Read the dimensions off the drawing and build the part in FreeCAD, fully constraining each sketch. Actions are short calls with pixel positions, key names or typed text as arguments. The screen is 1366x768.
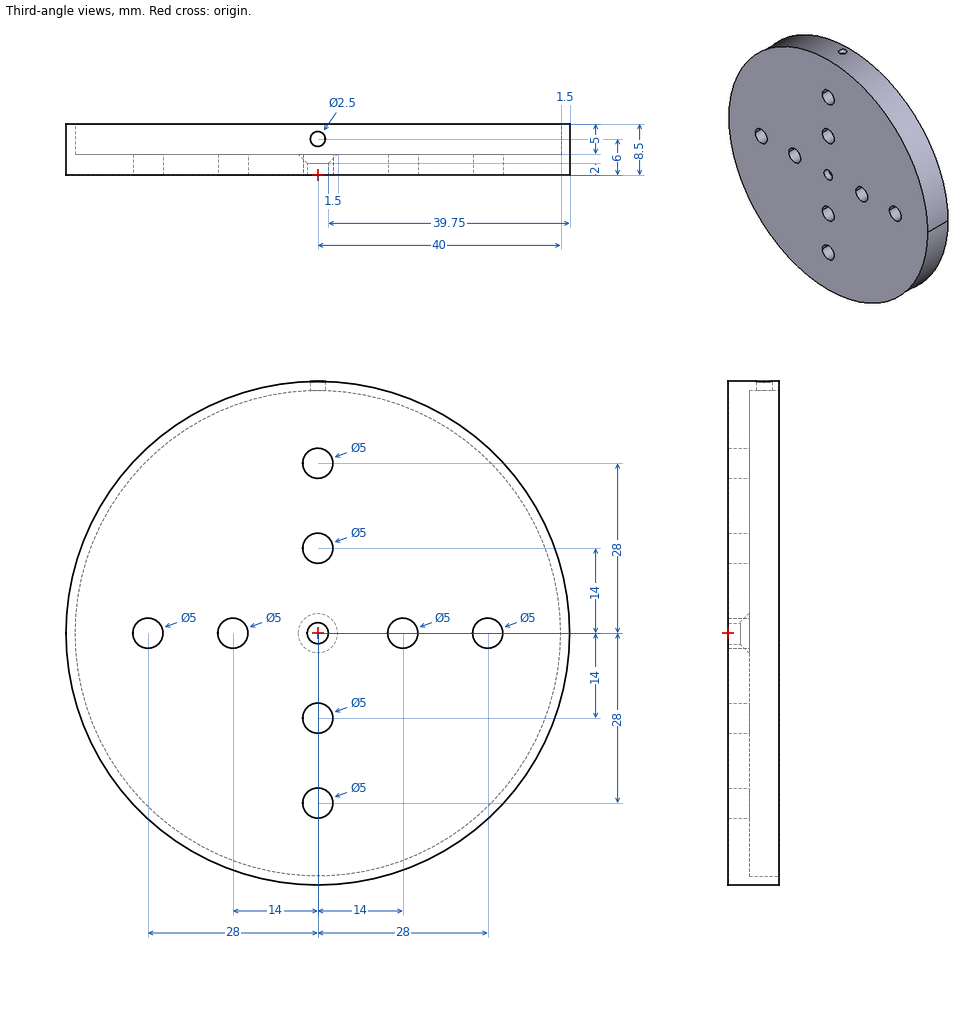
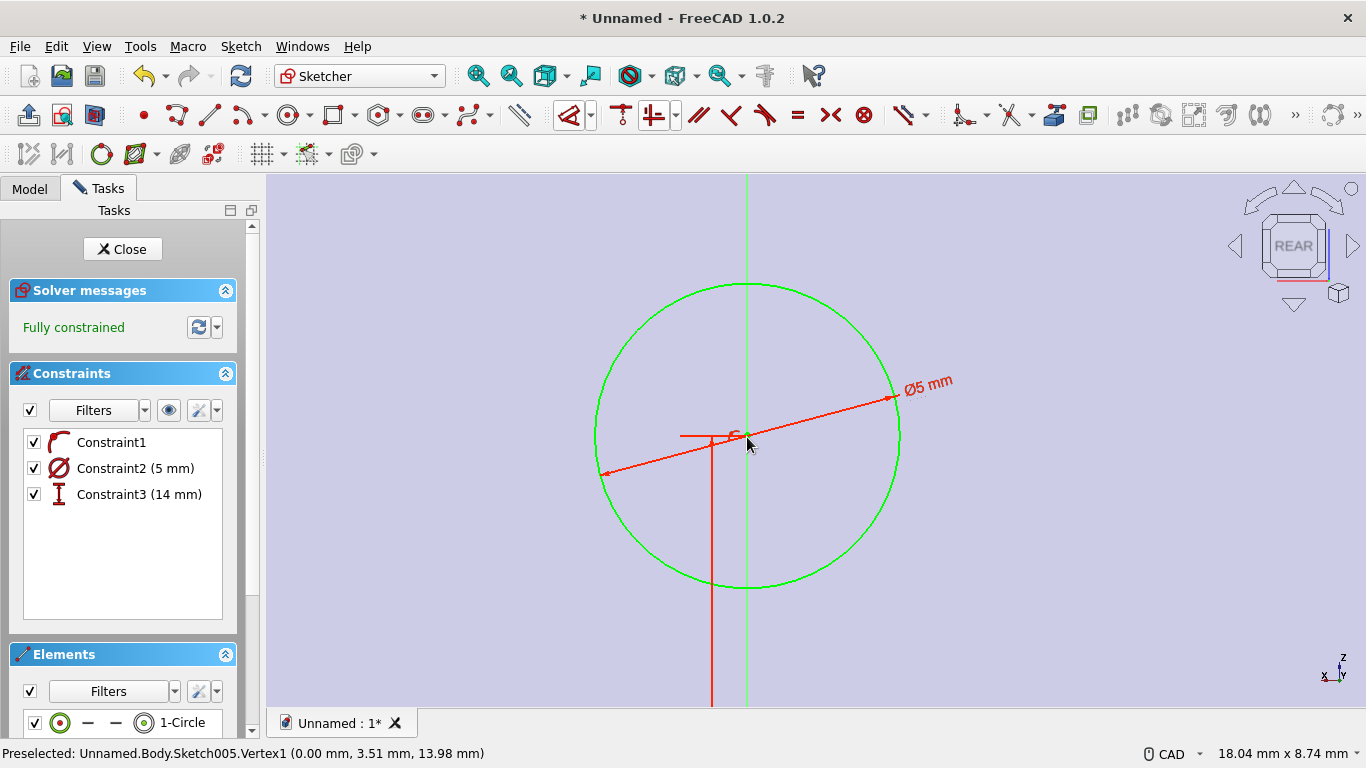
click(123, 249)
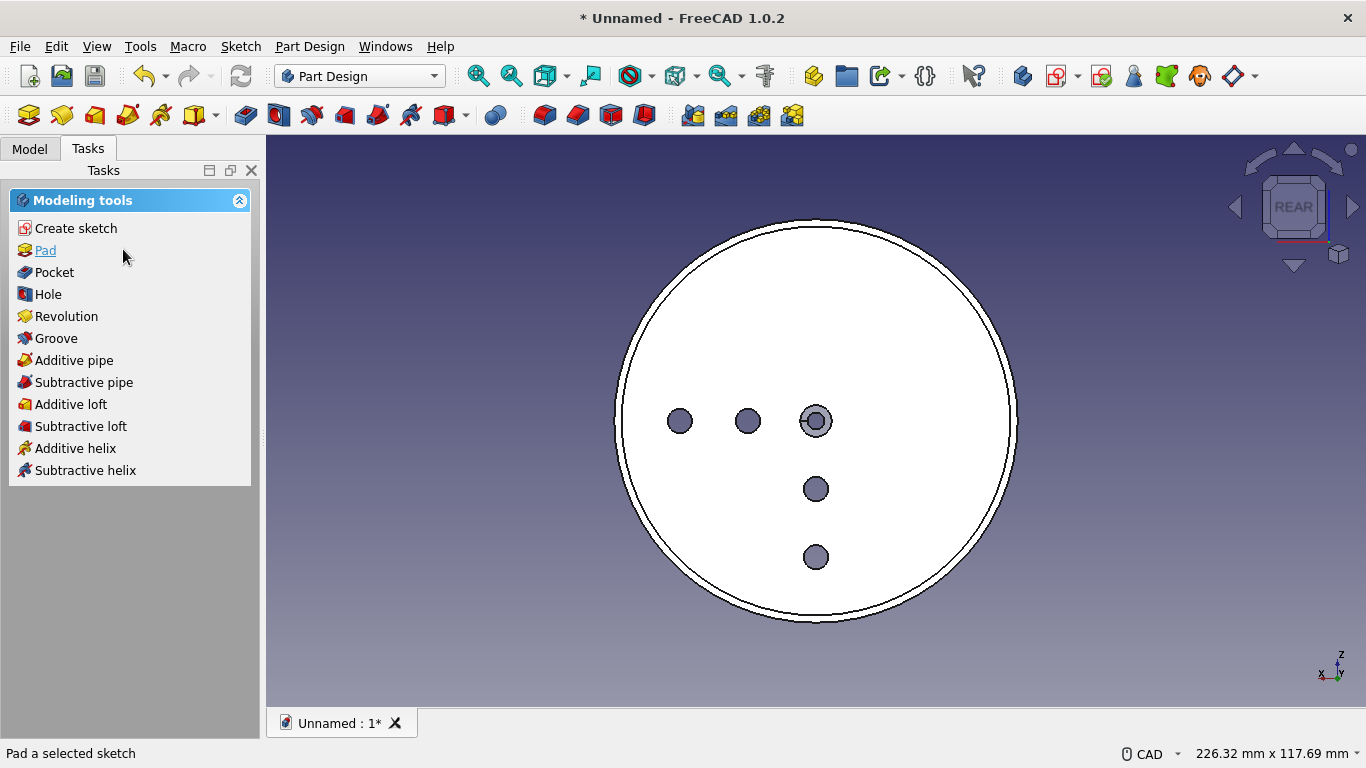
click(246, 116)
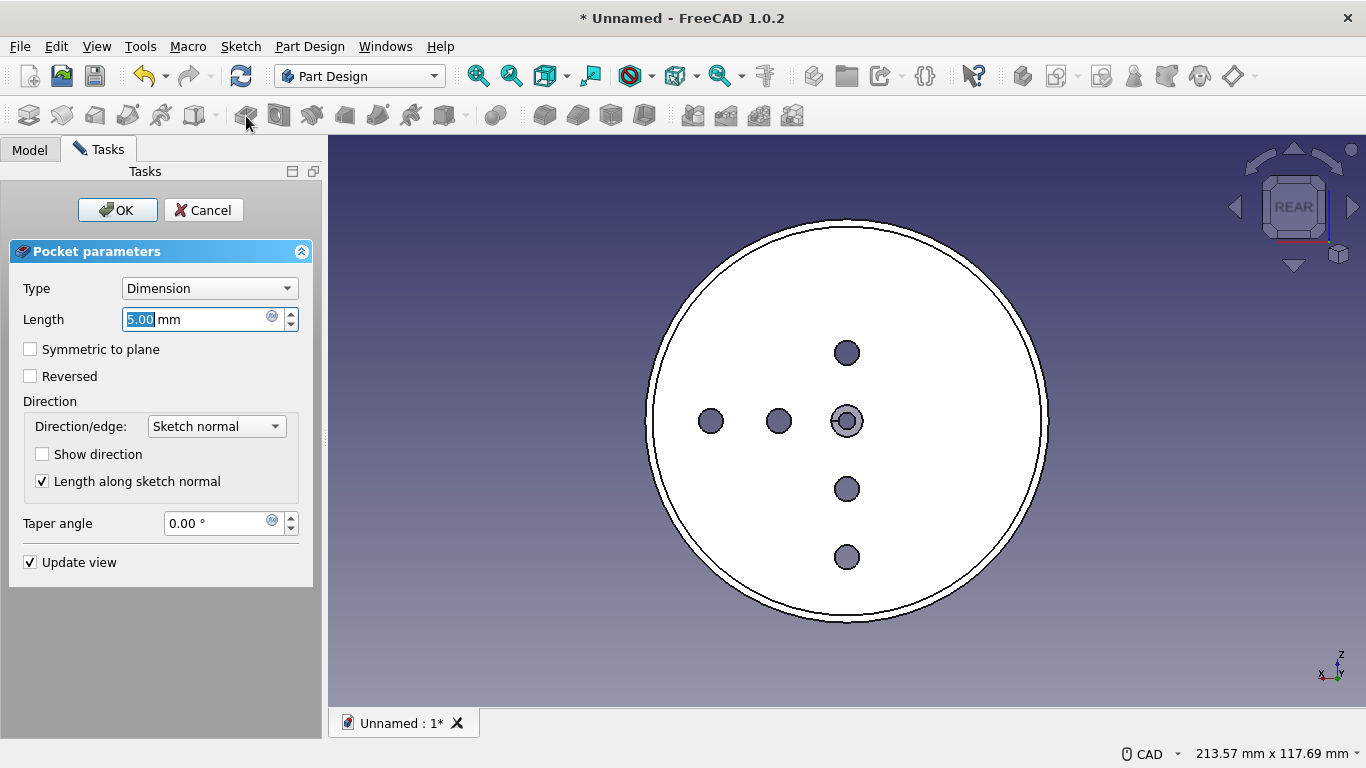
click(210, 288)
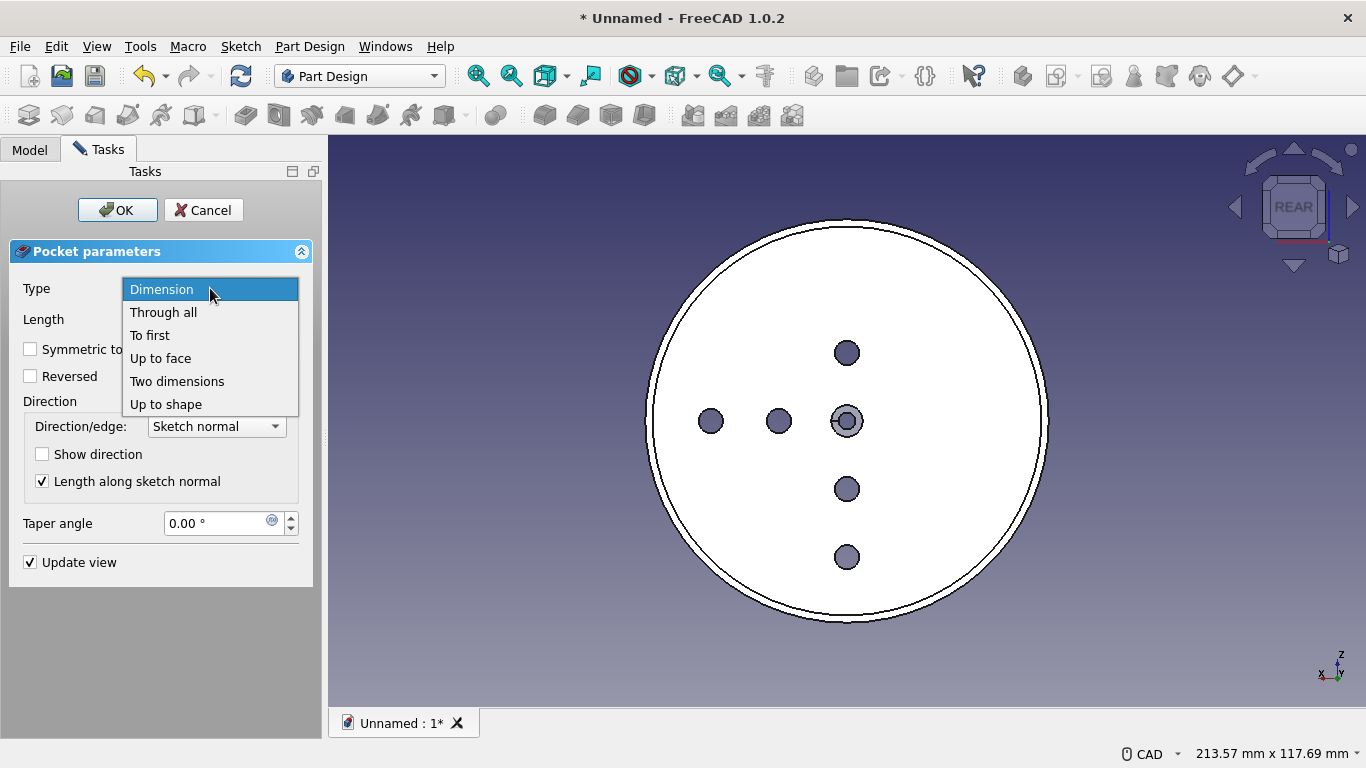
click(208, 336)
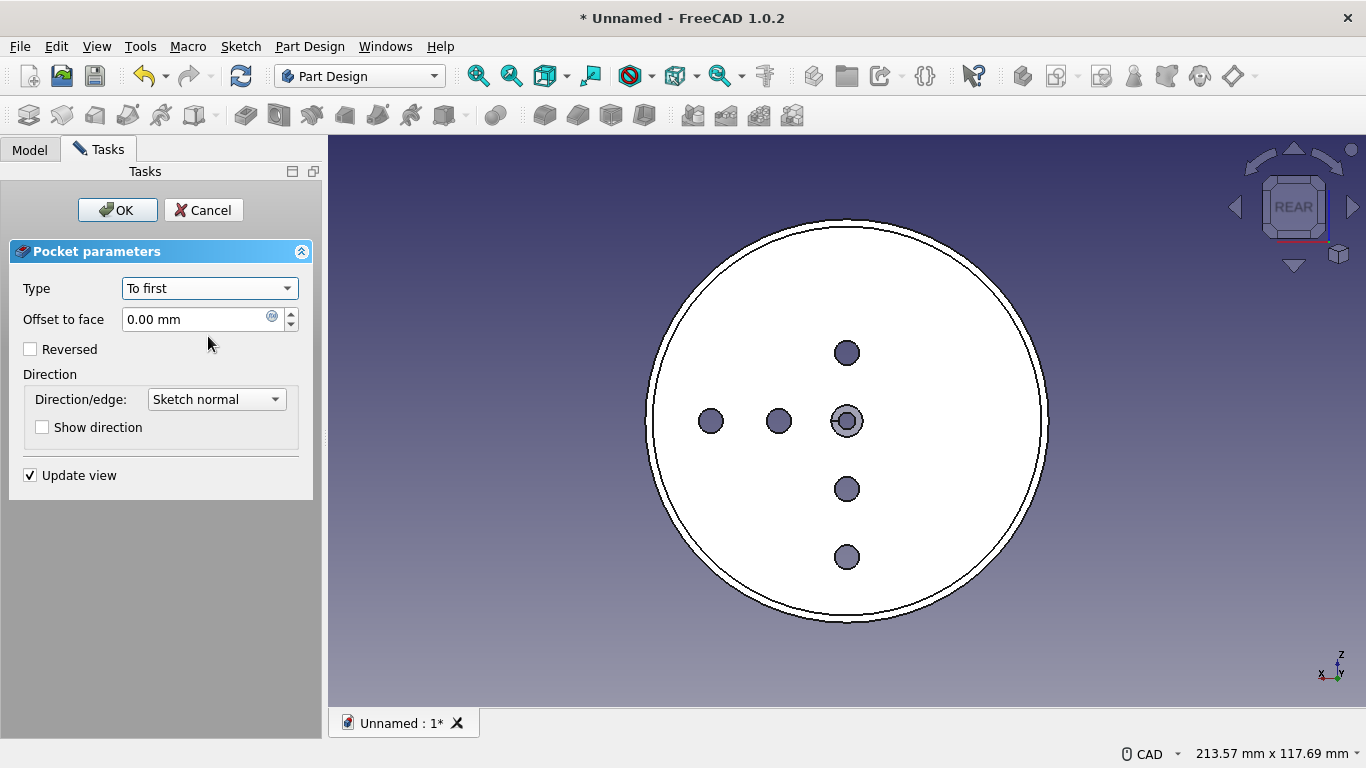
click(118, 210)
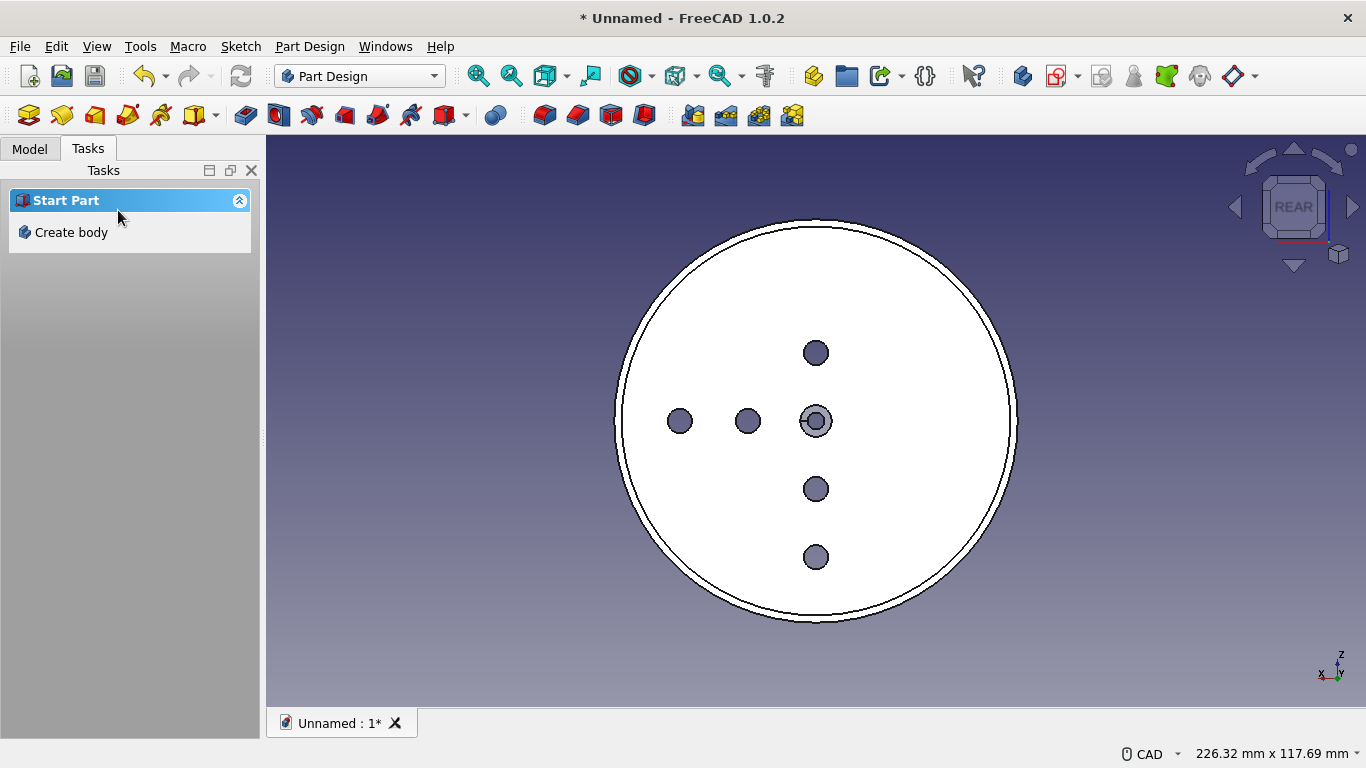
click(927, 420)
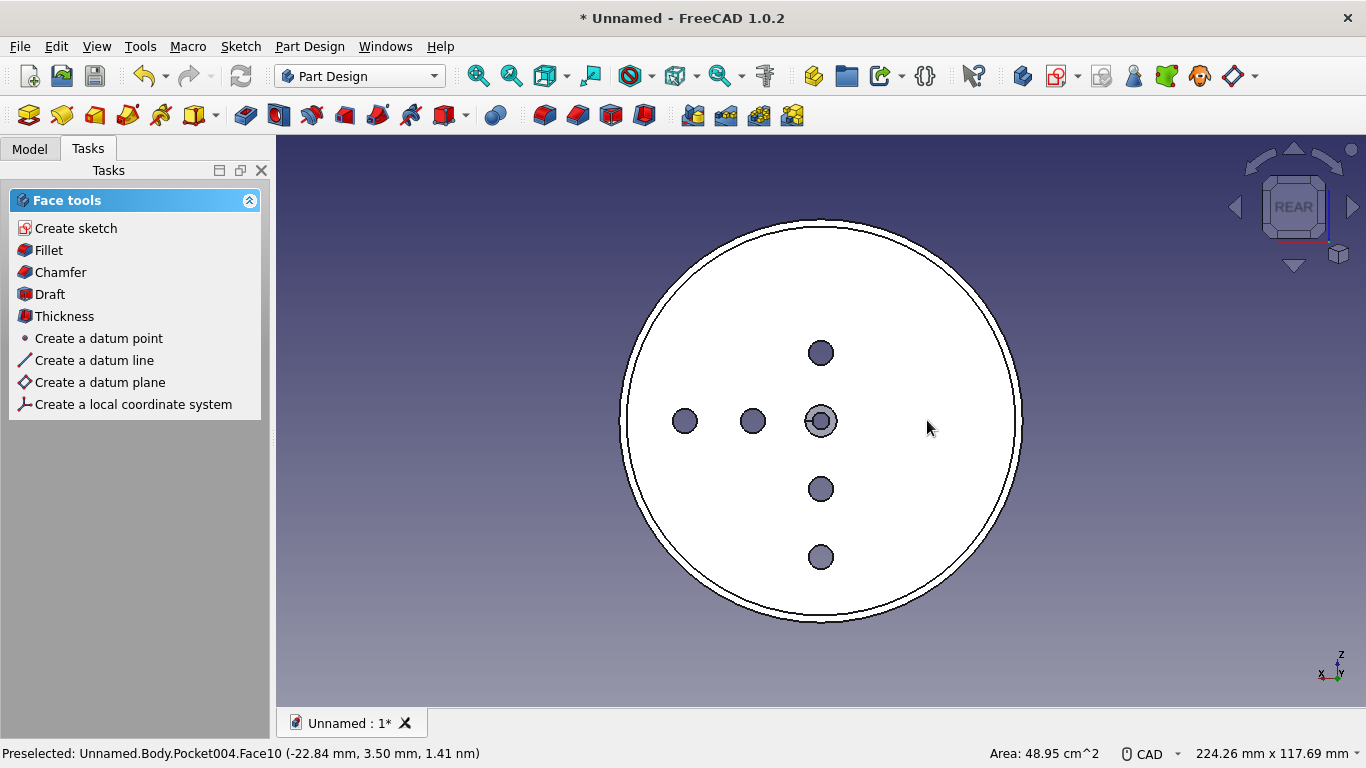
click(1056, 76)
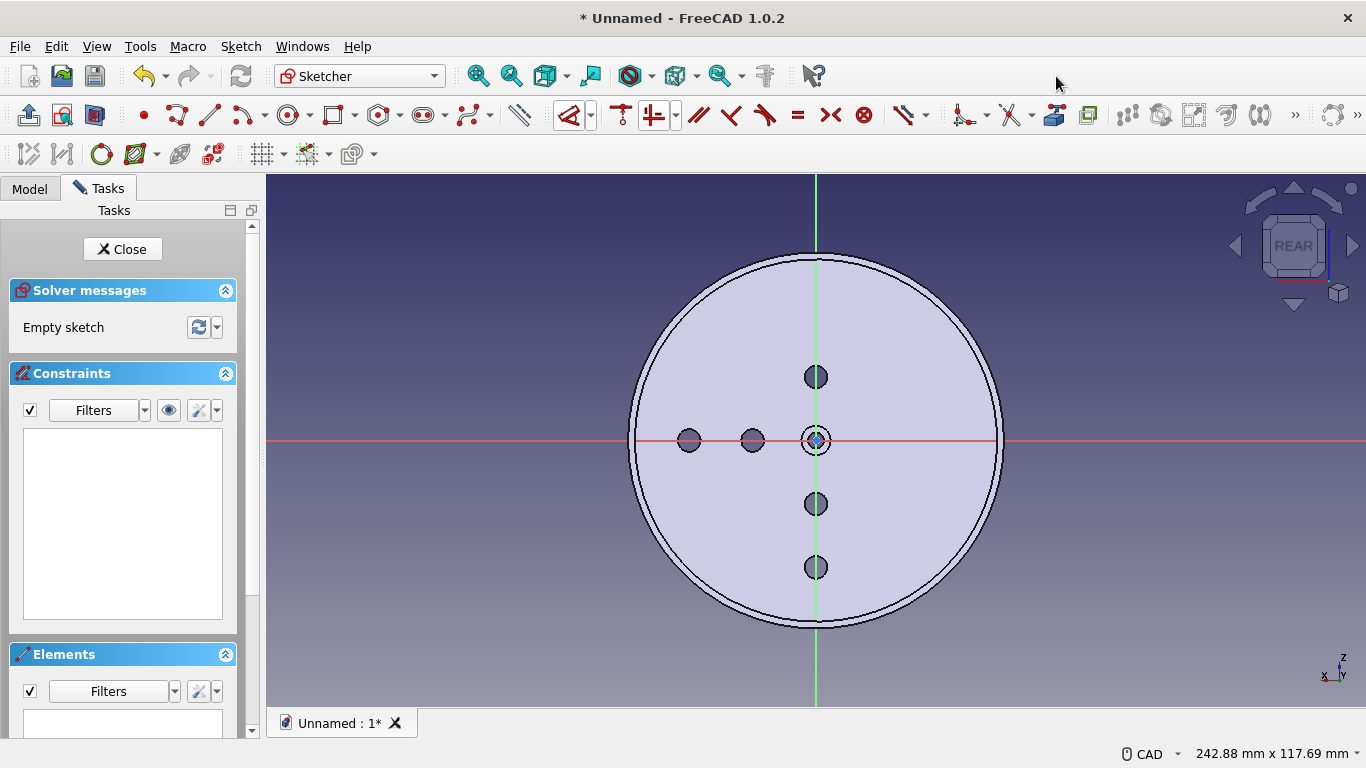
scroll(821, 304, up, 13)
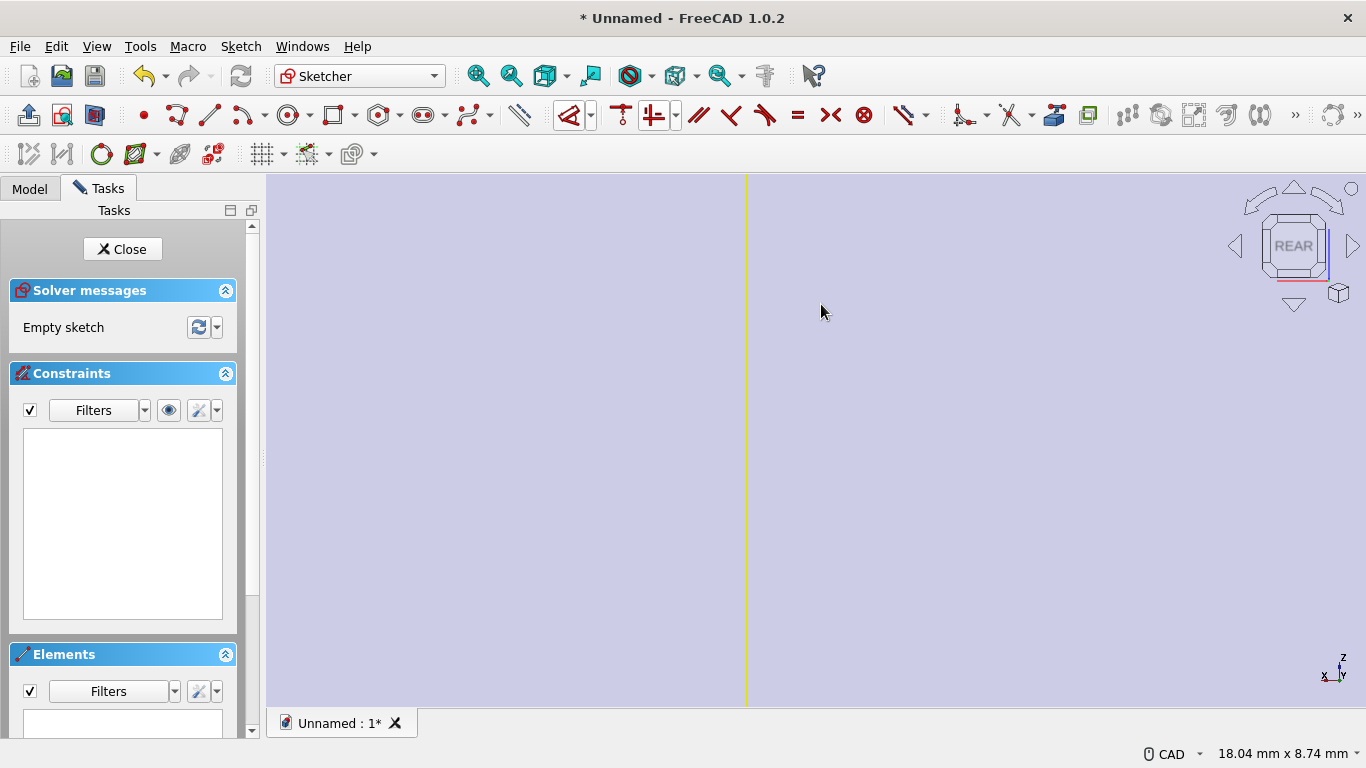
click(288, 116)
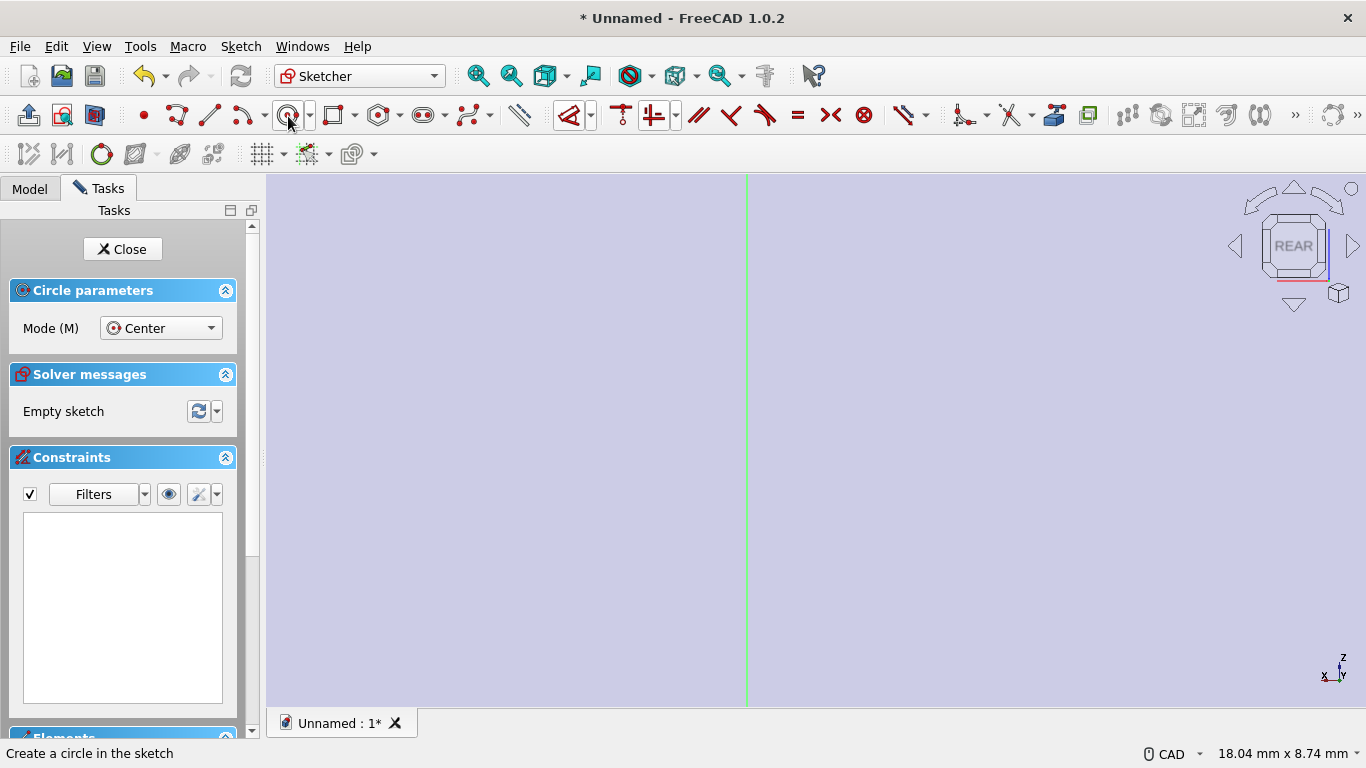
click(747, 431)
click(855, 324)
key(Escape)